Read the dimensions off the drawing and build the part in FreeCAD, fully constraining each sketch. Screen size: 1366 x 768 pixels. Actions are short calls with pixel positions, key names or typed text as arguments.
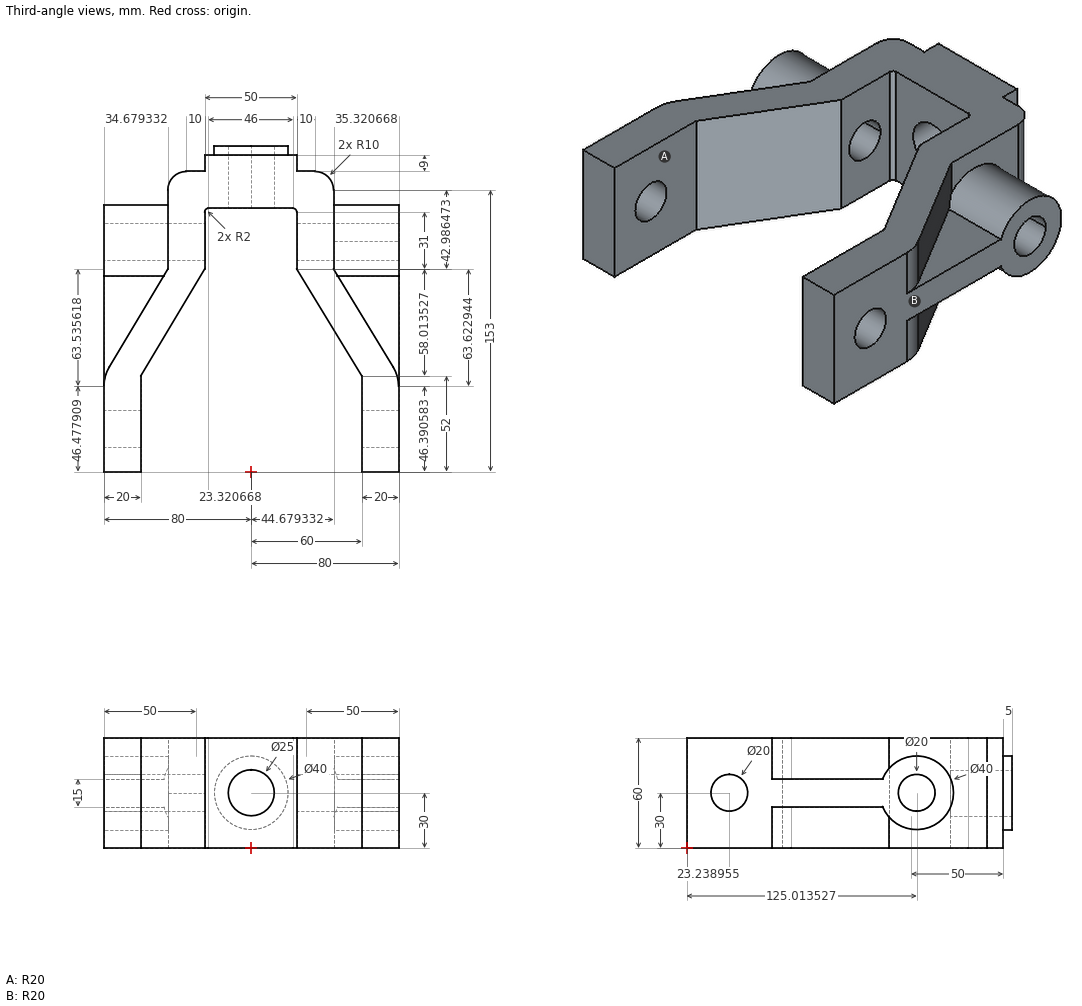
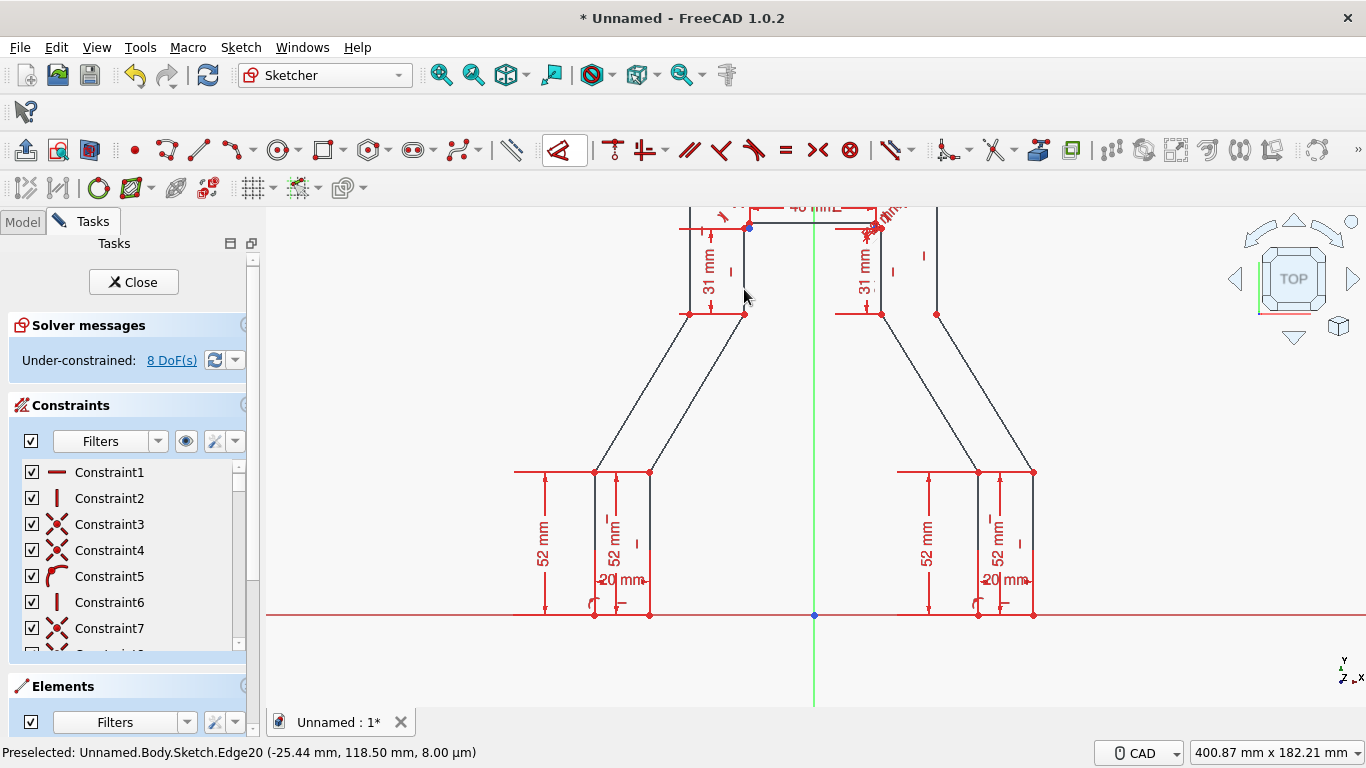
click(978, 472)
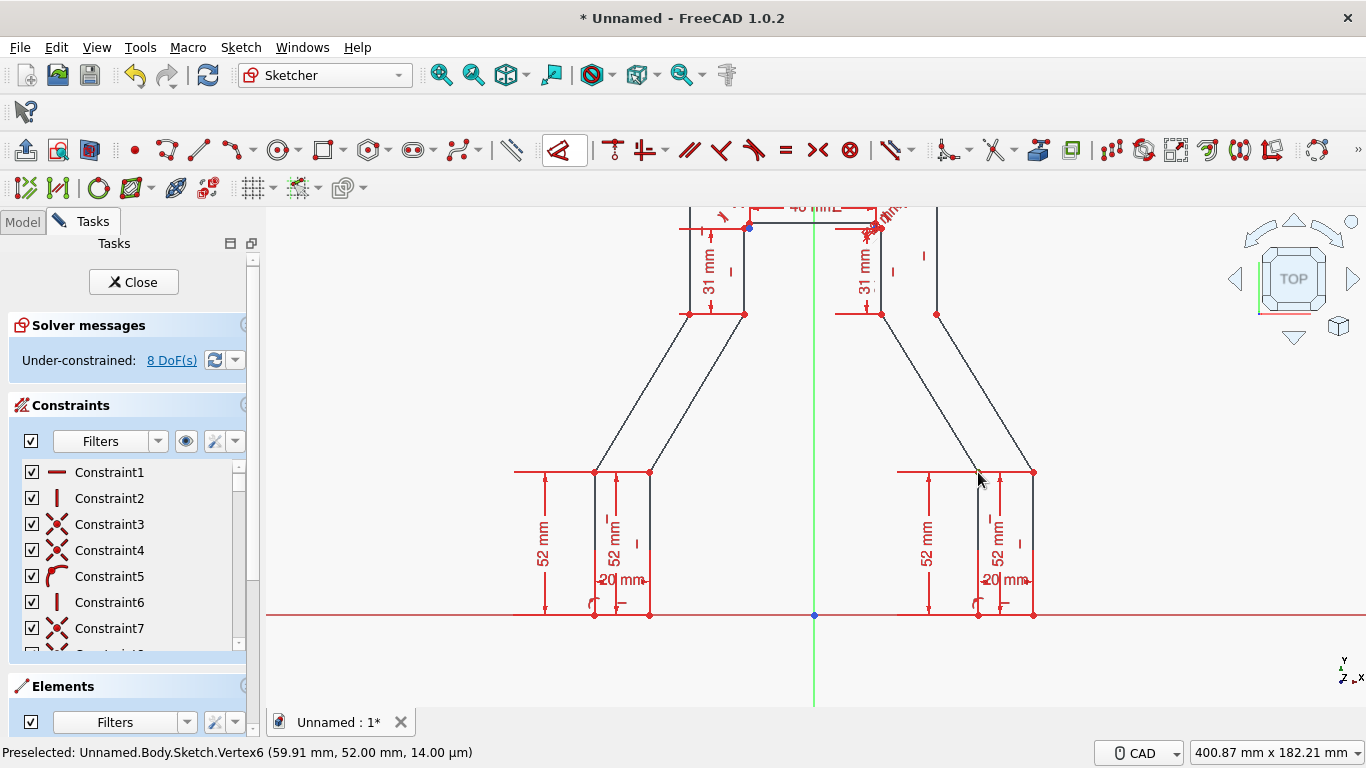
key(l)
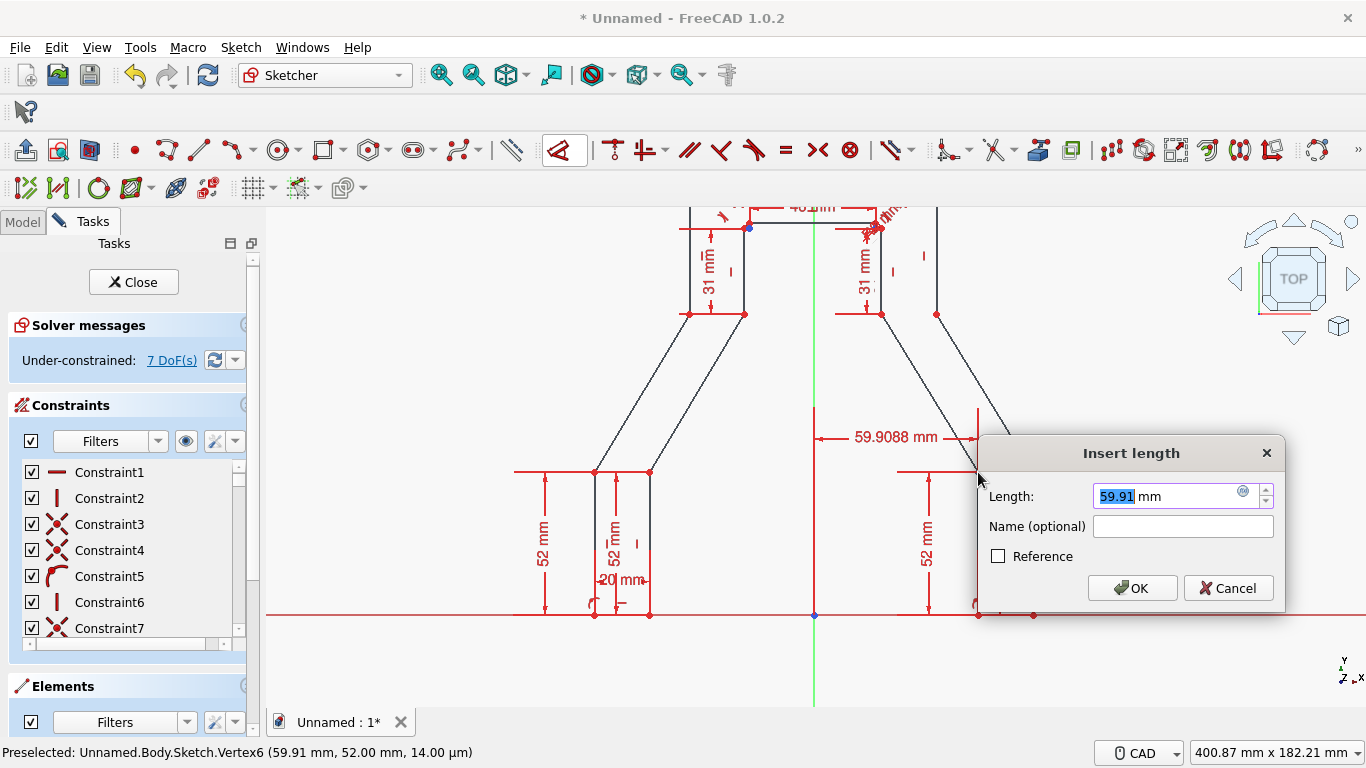
text(60)
key(Return)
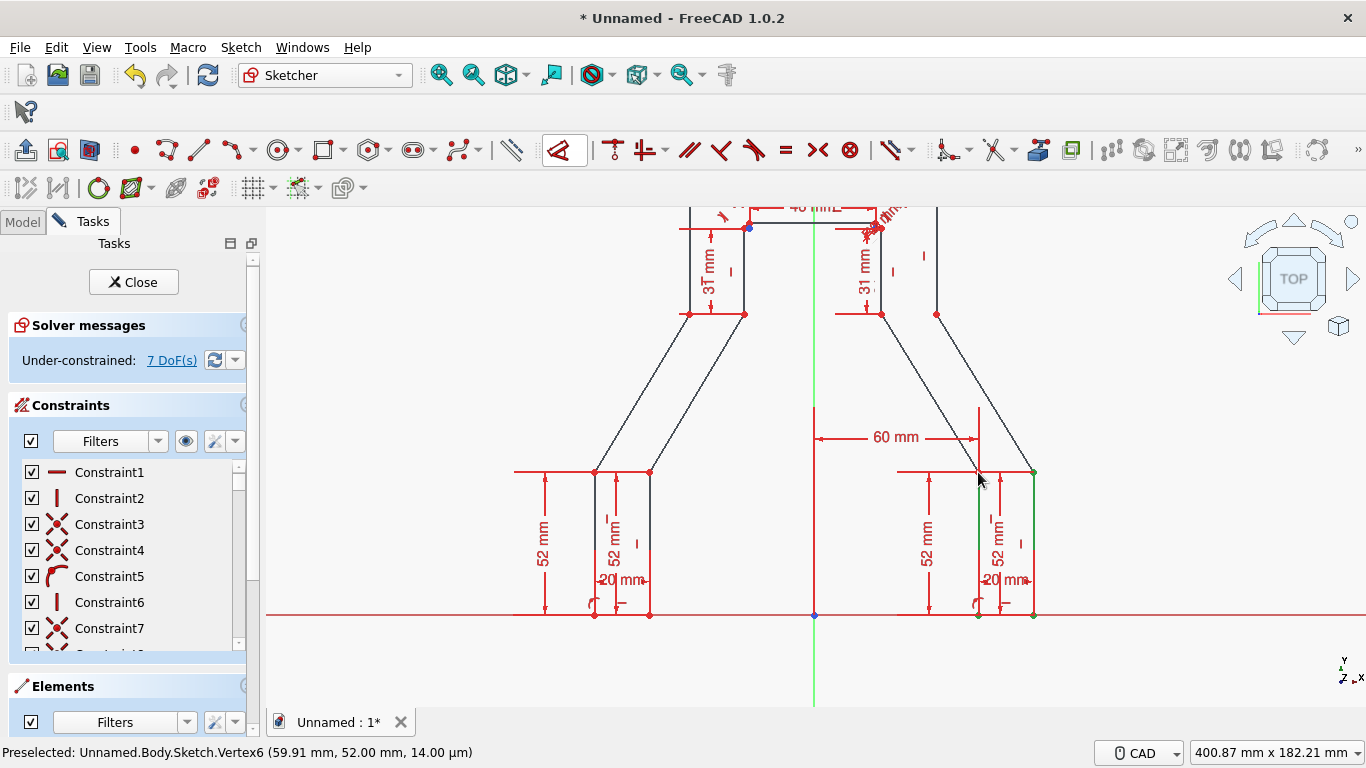
click(595, 472)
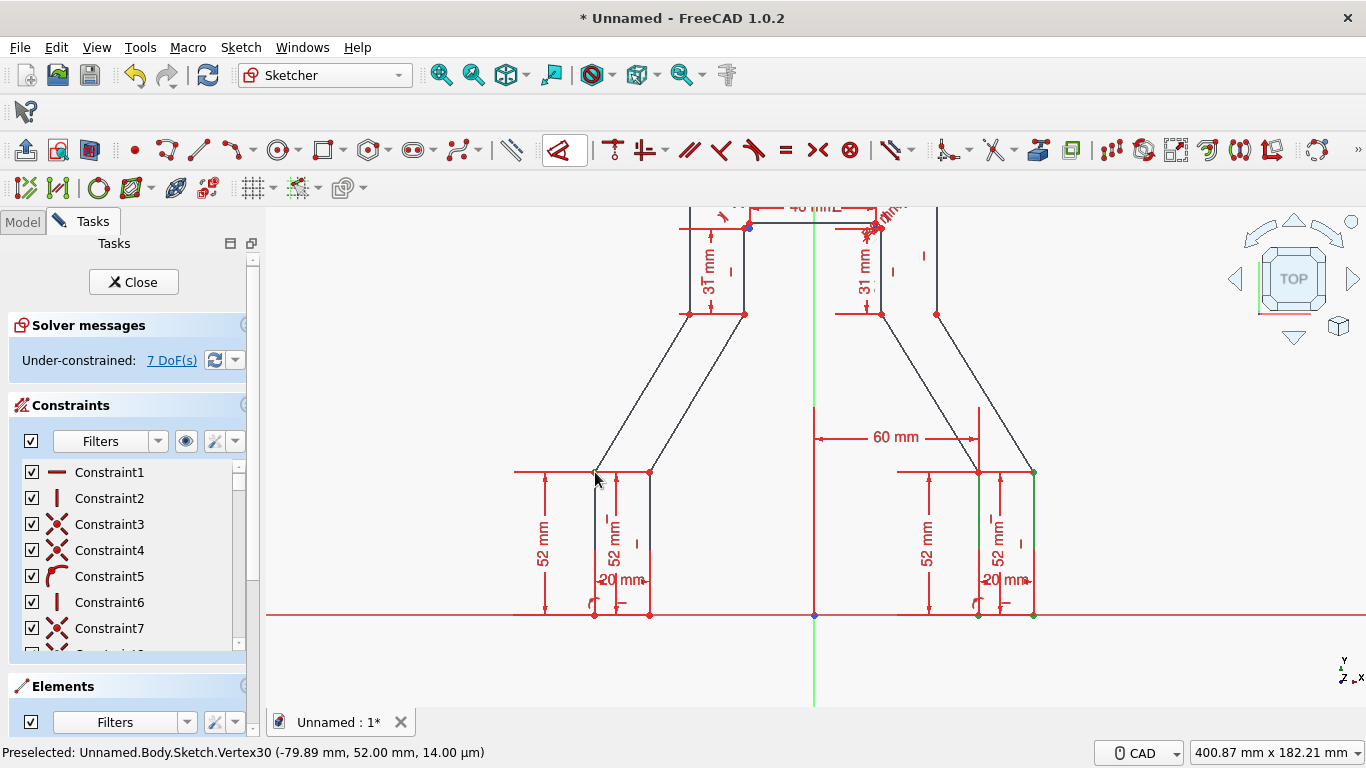
key(l)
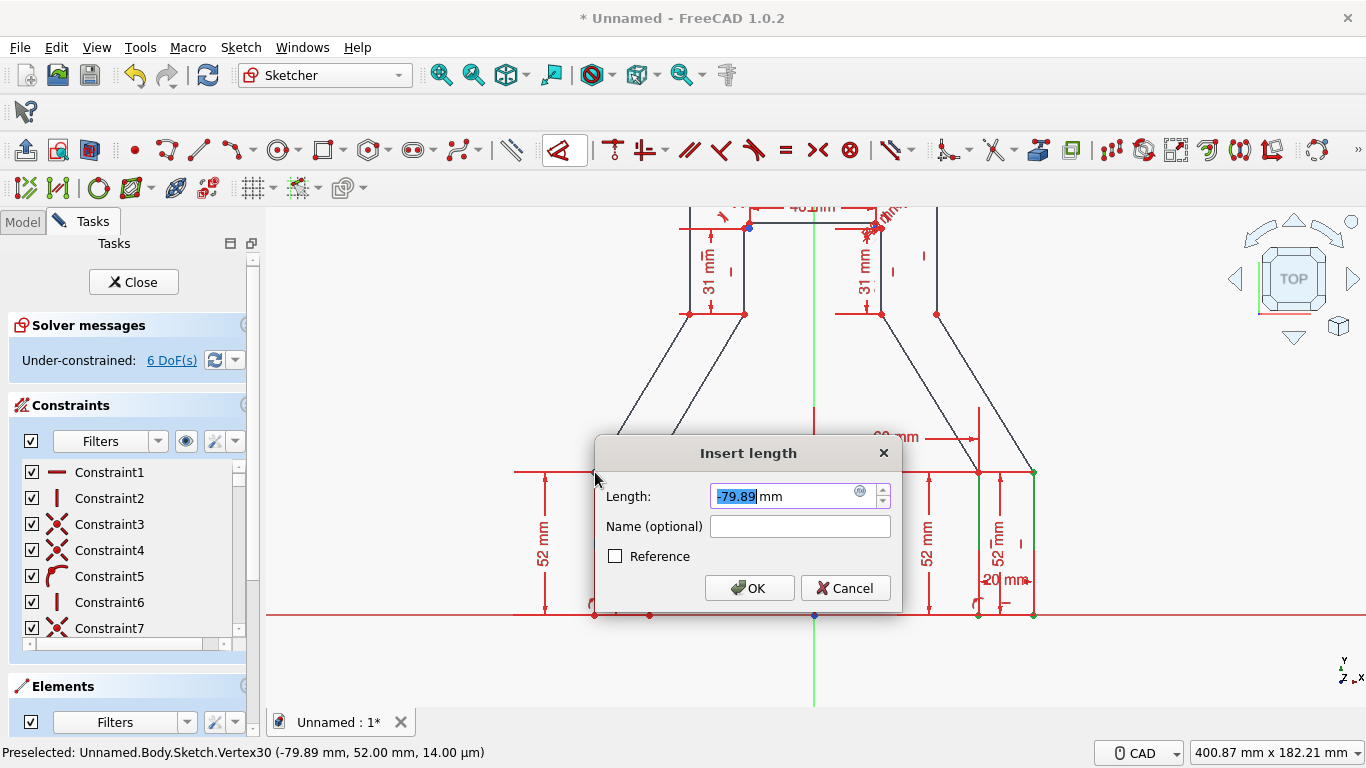
text(-80)
key(Return)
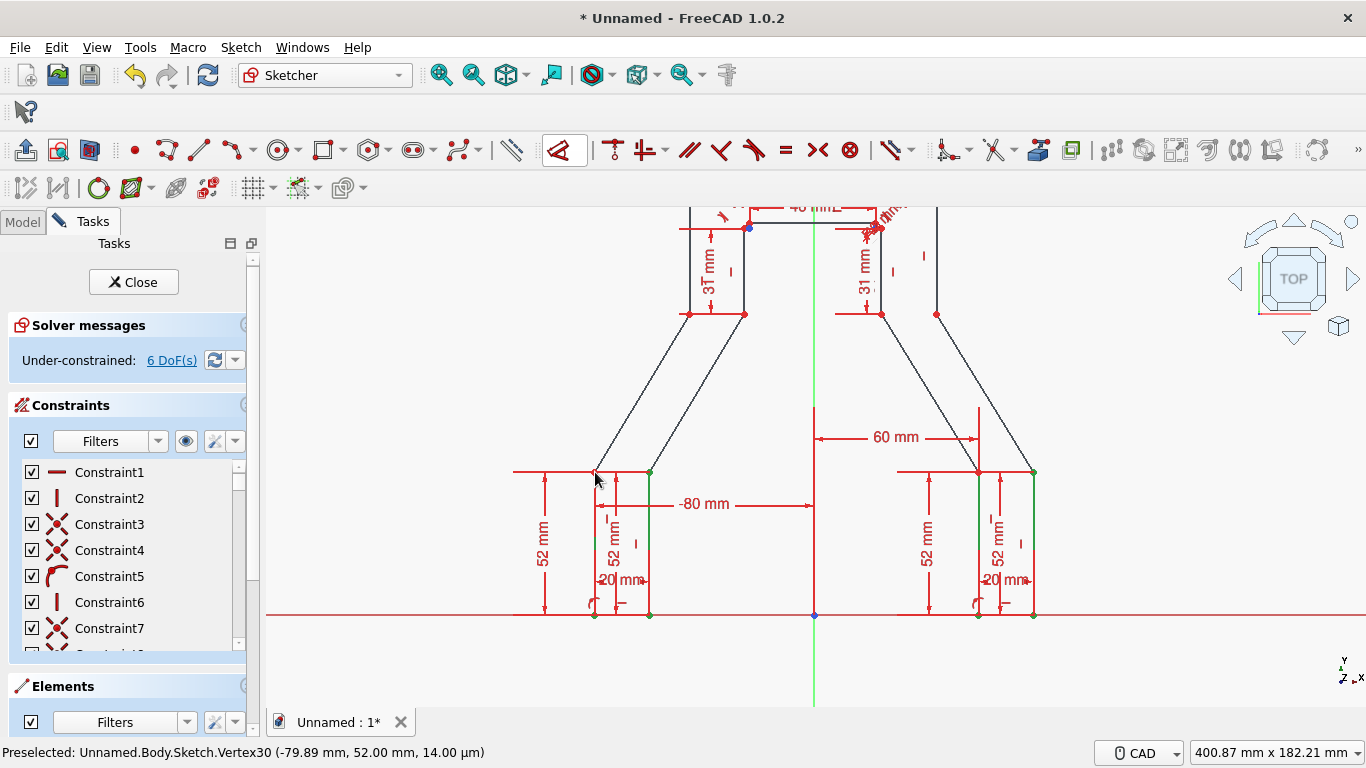
scroll(612, 615, down, 2)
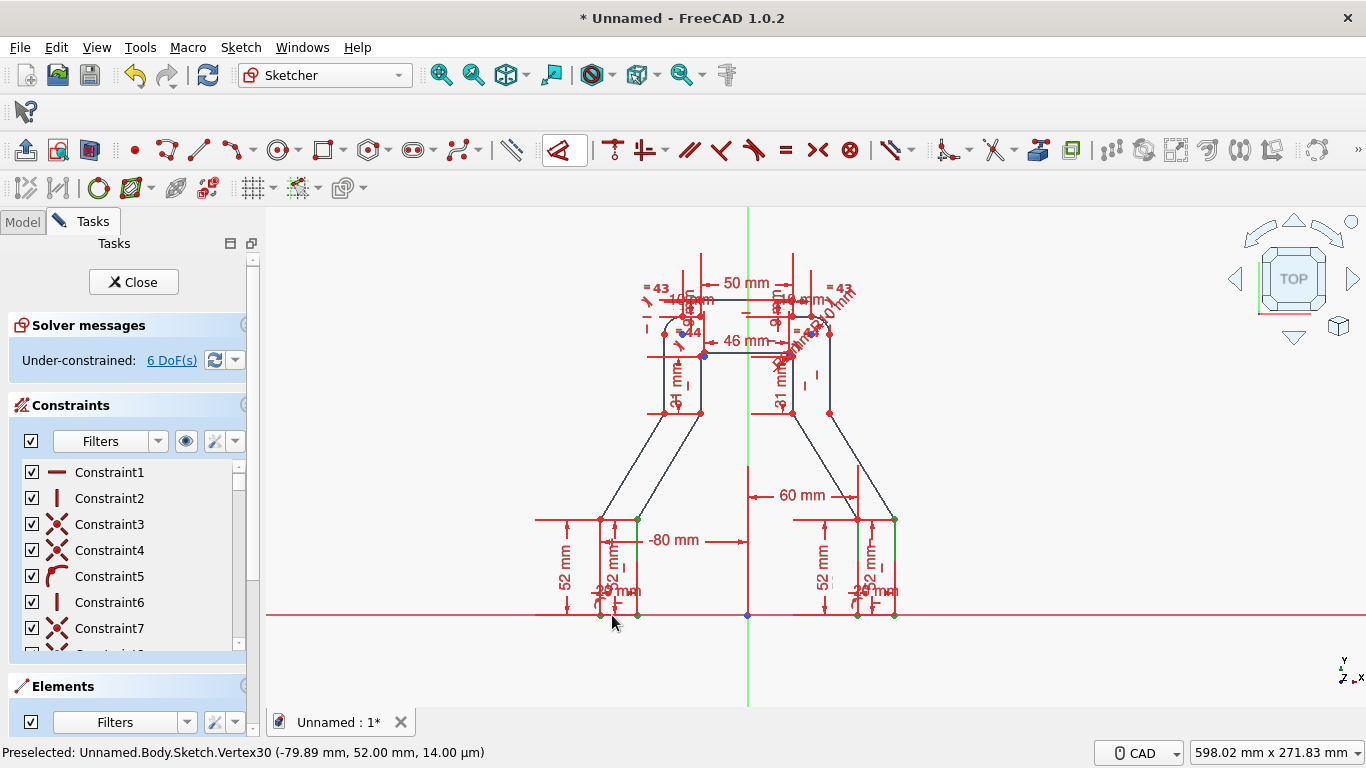
click(830, 335)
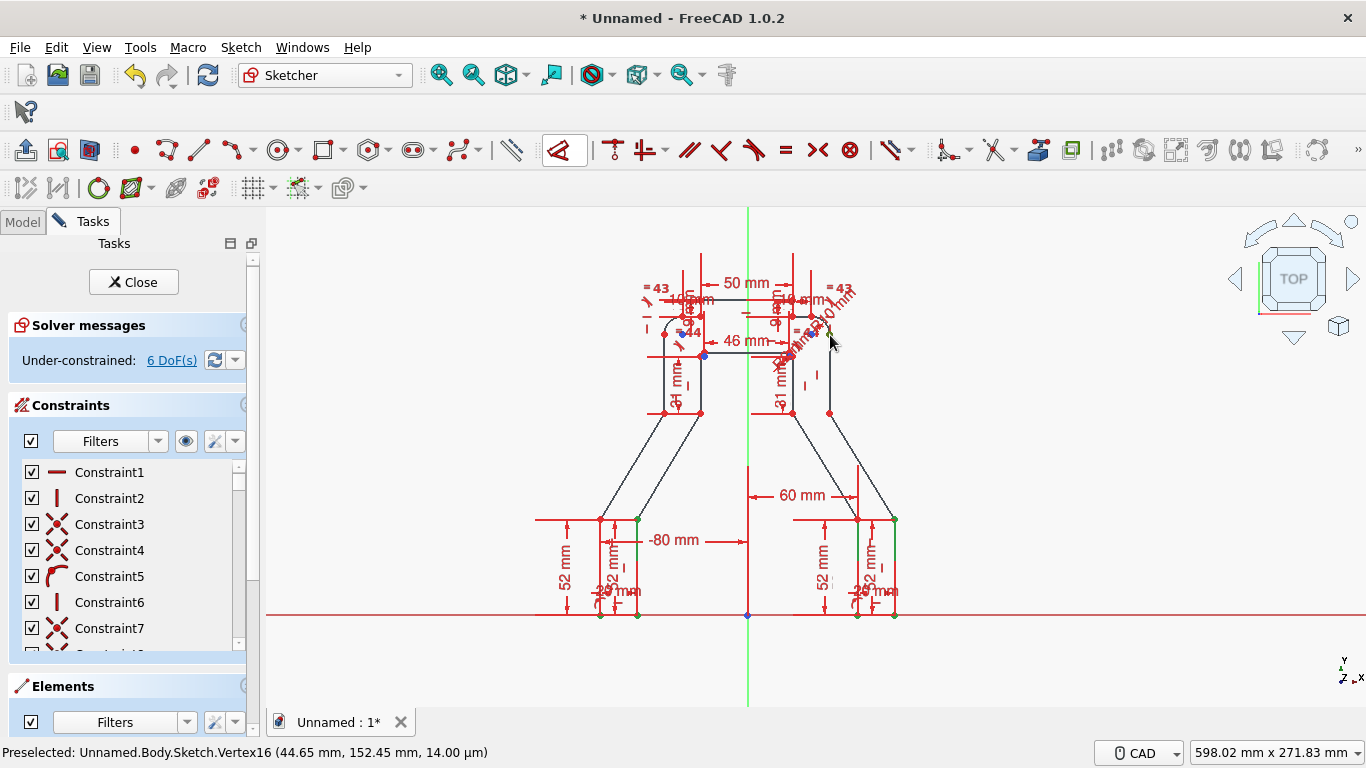
key(i)